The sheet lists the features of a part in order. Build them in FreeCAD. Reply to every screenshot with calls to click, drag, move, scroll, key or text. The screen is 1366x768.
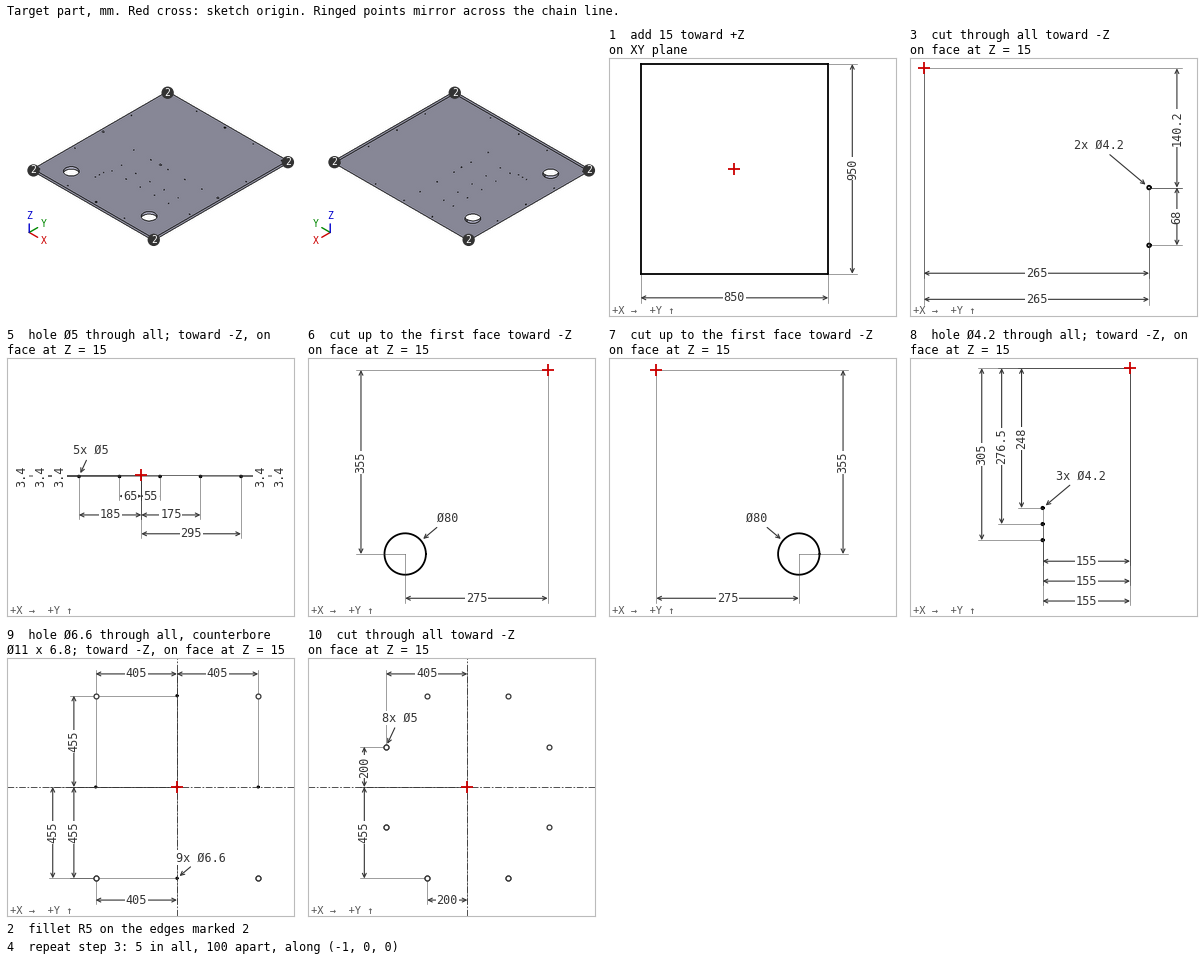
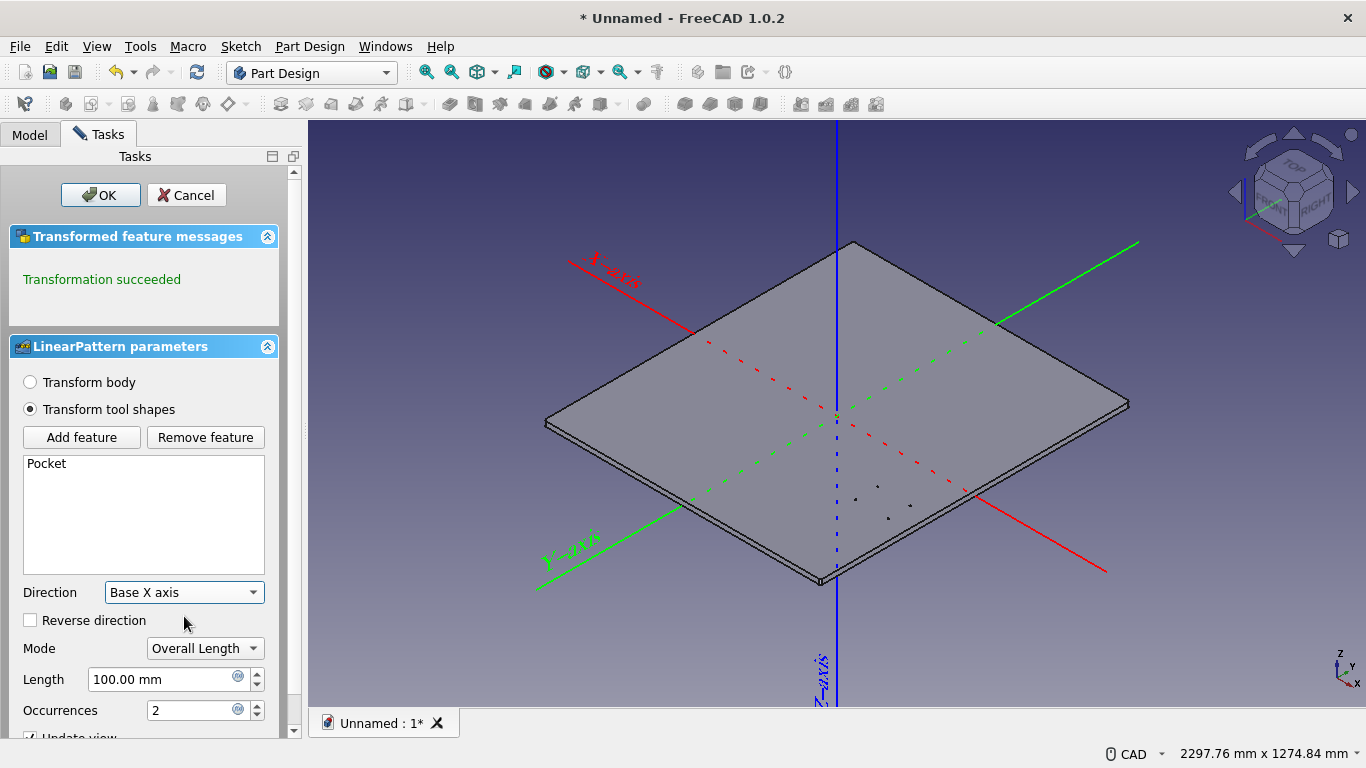
click(206, 648)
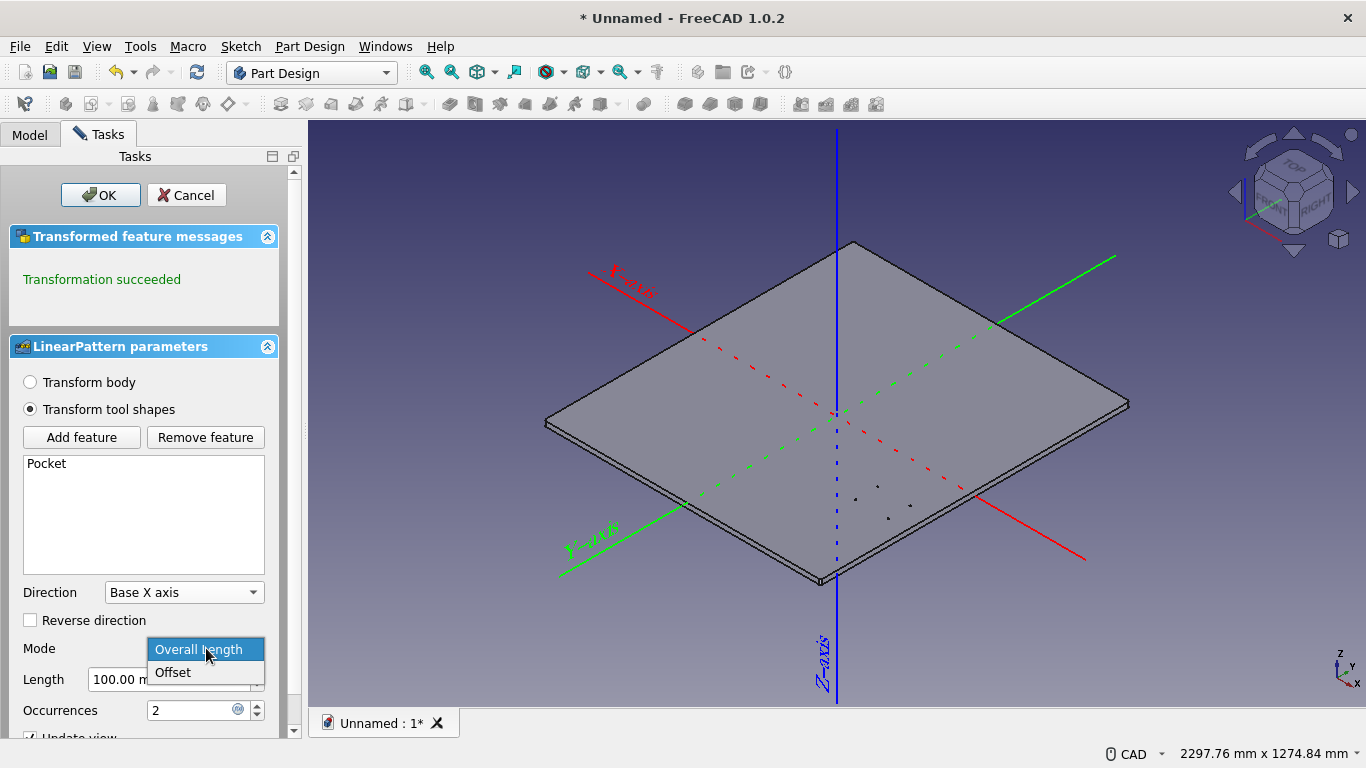
click(204, 672)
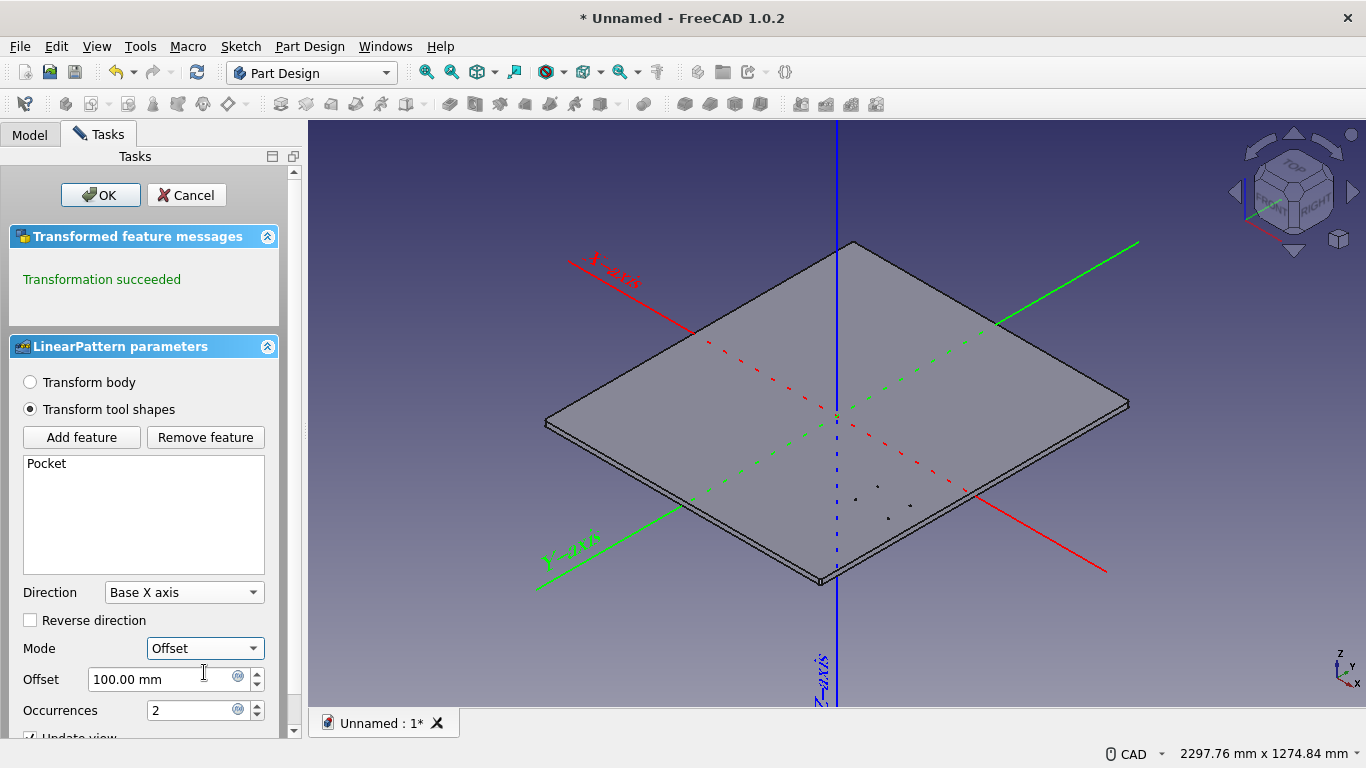
triple_click(170, 680)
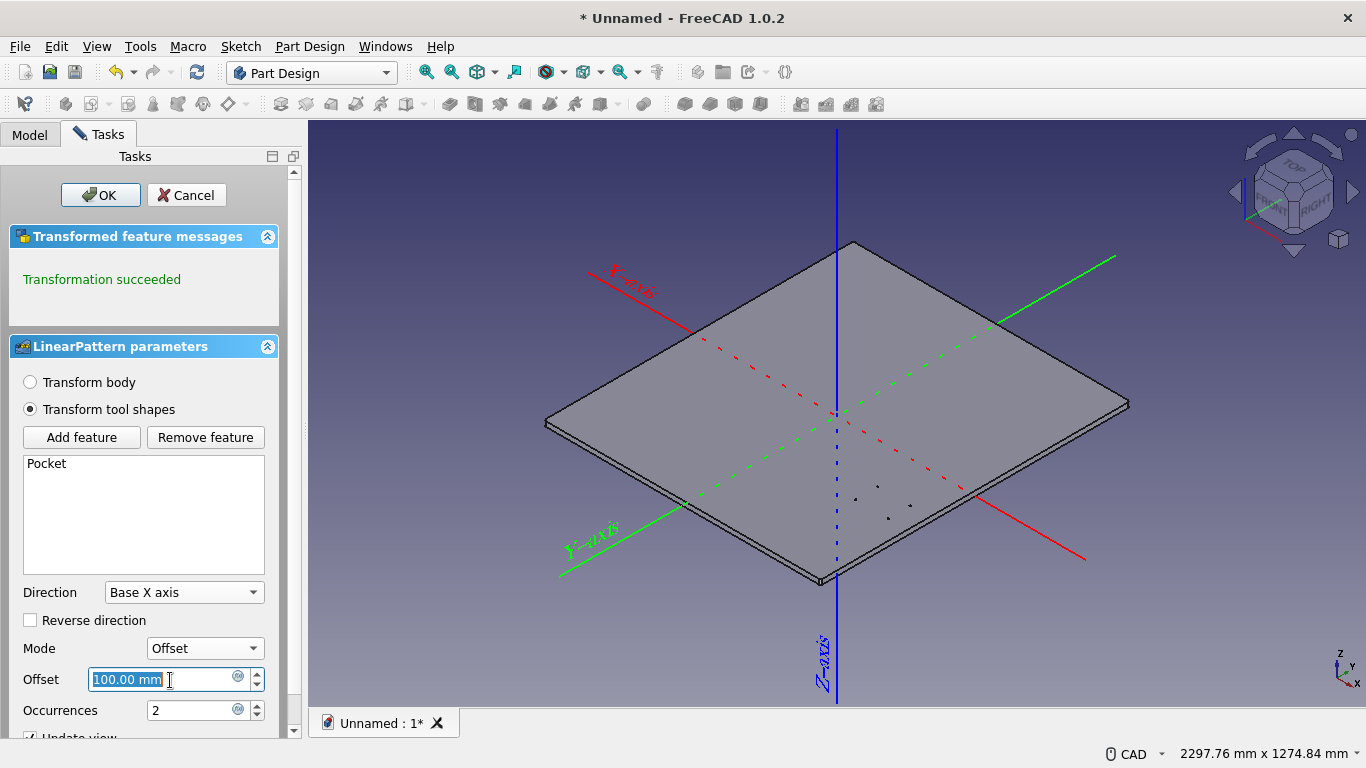
text(100)
key(Tab)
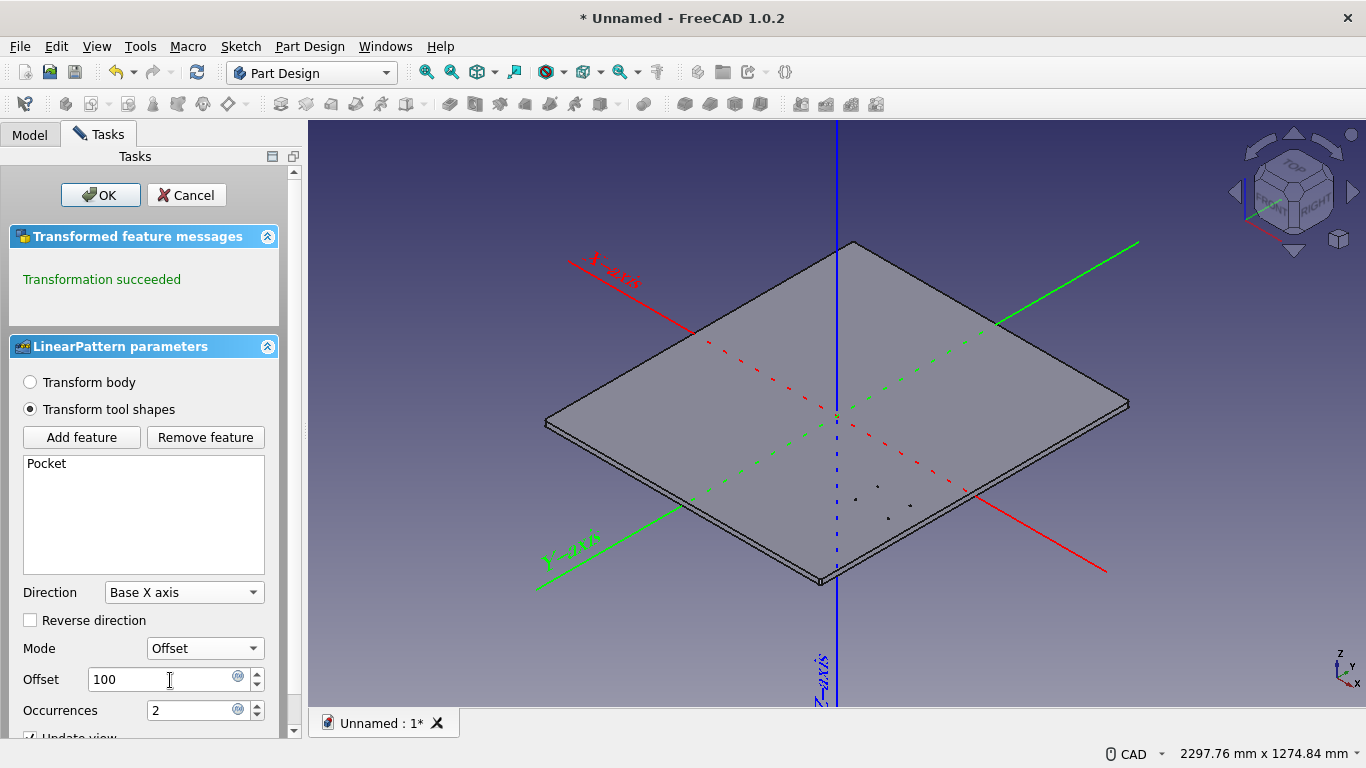
triple_click(199, 710)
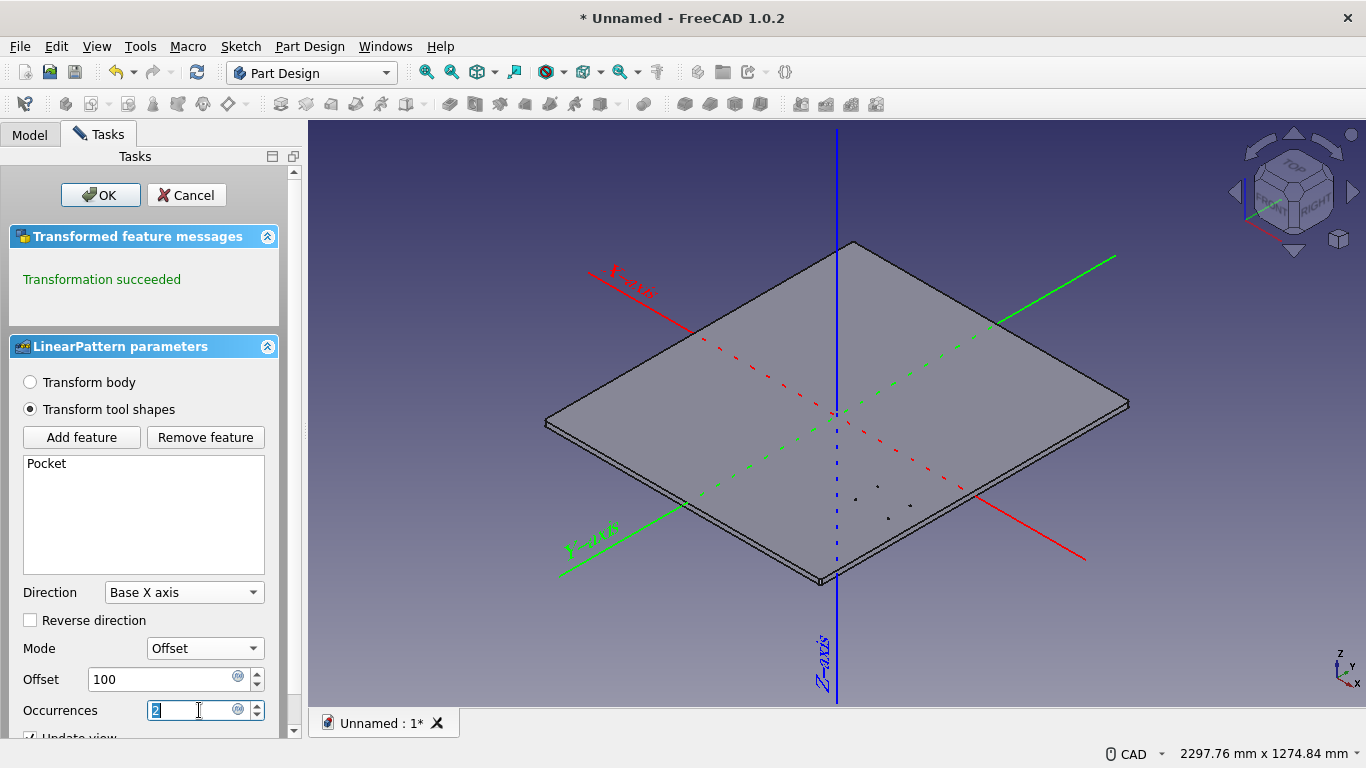
text(5)
key(Tab)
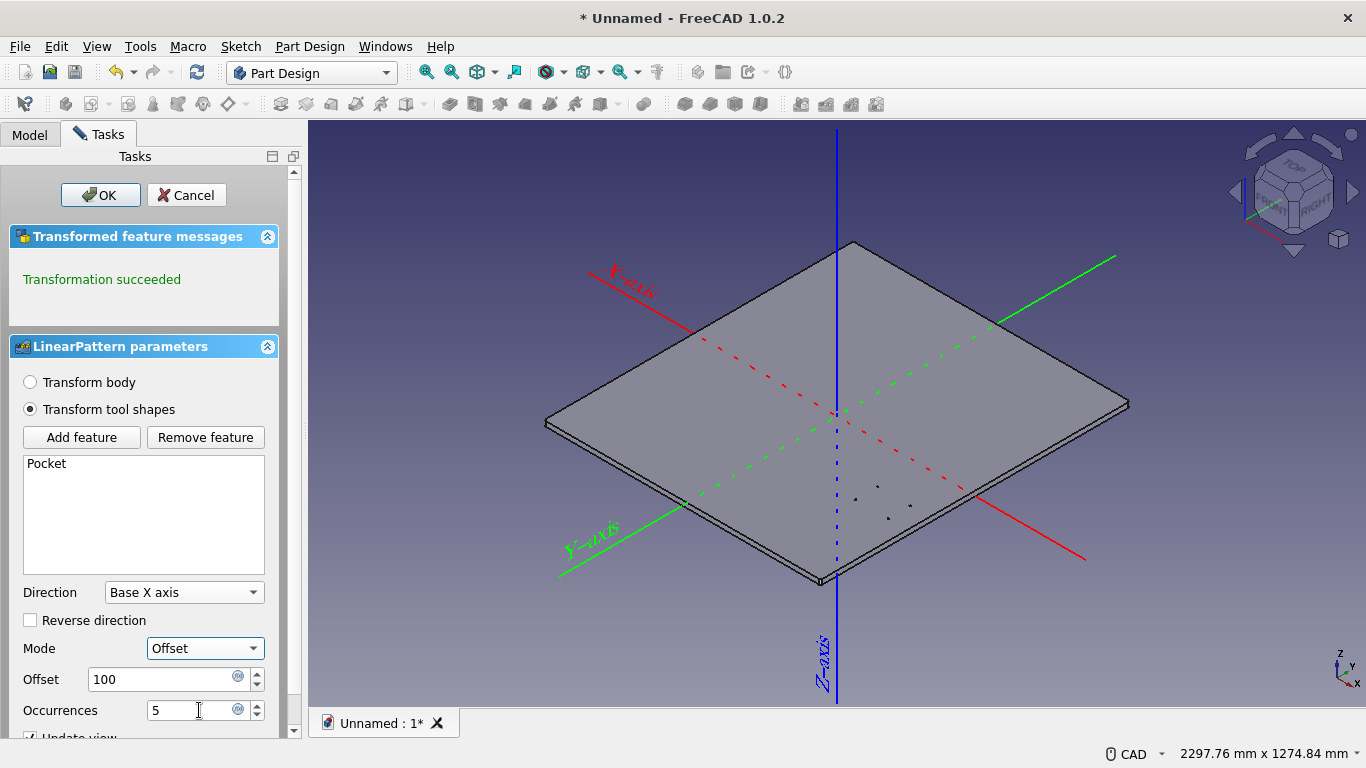
click(31, 620)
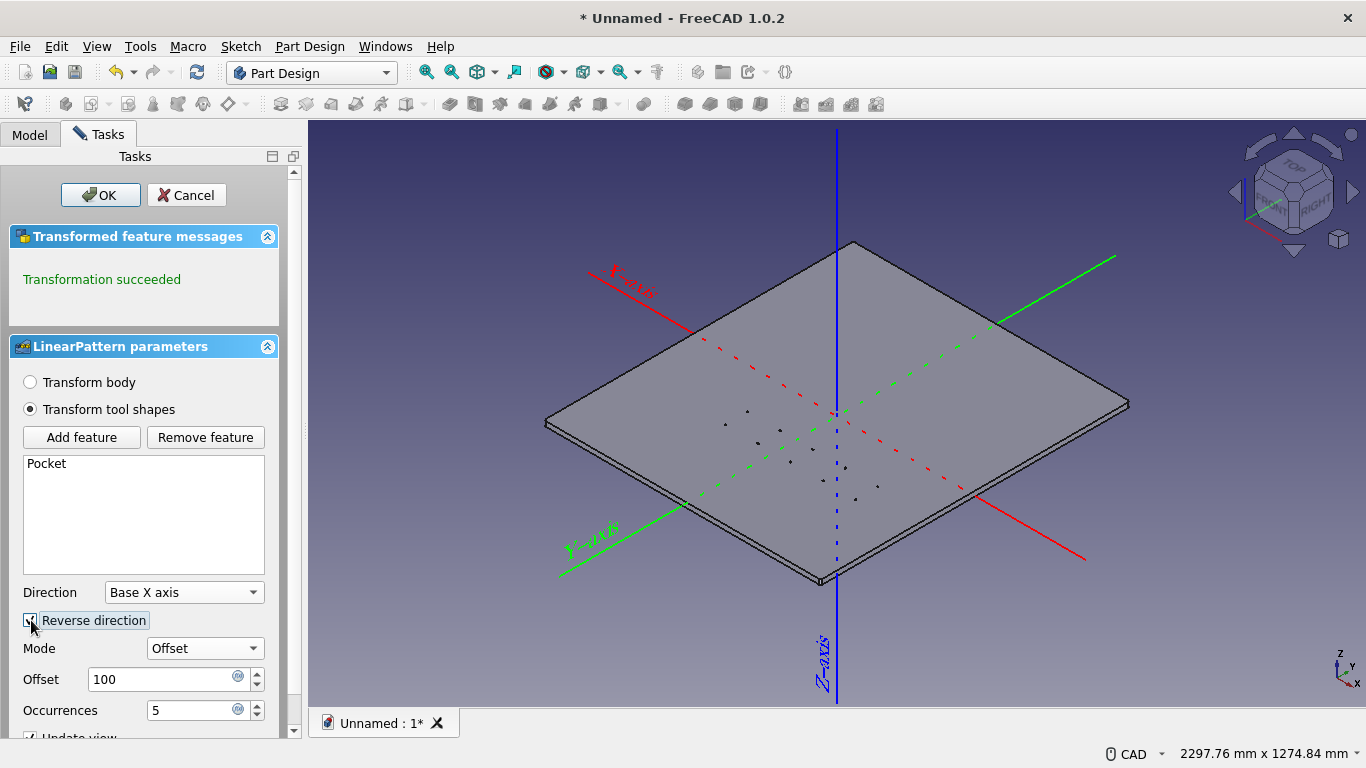
click(101, 195)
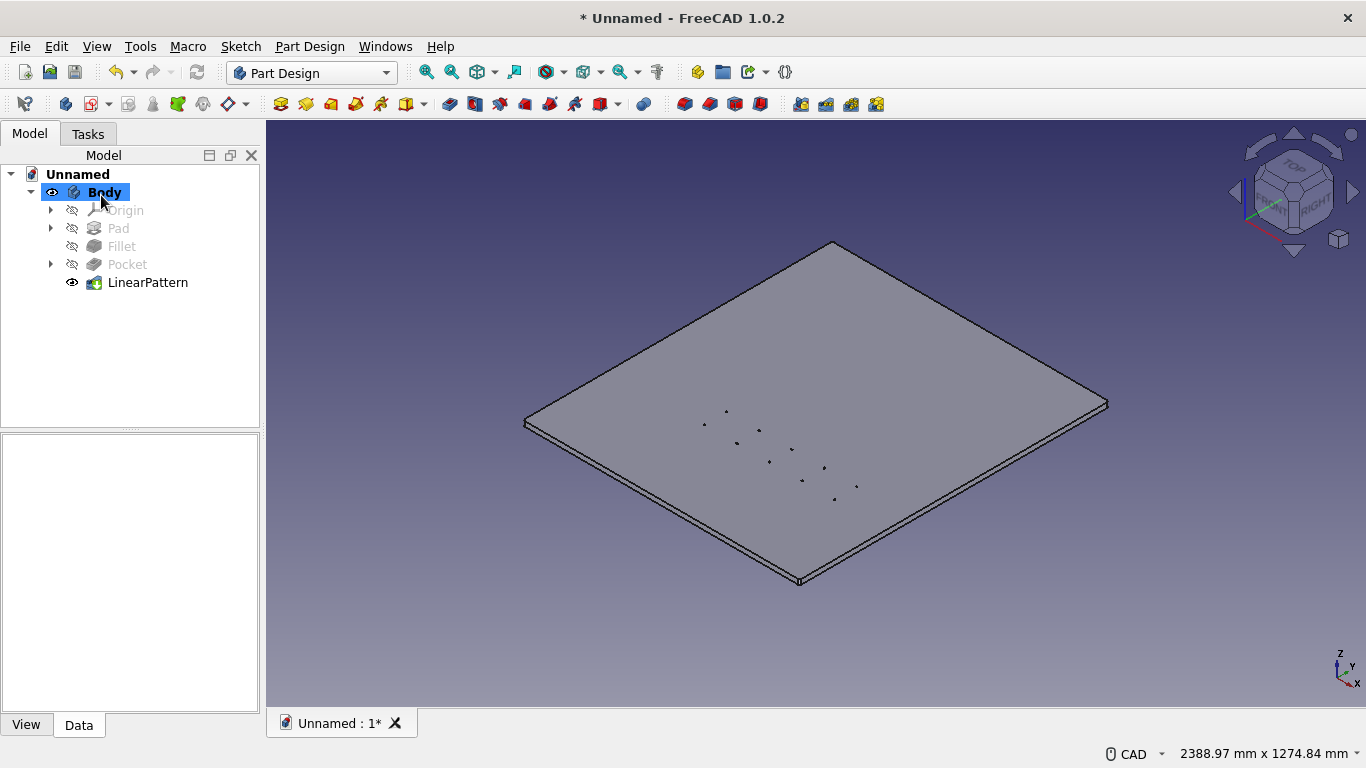
click(900, 407)